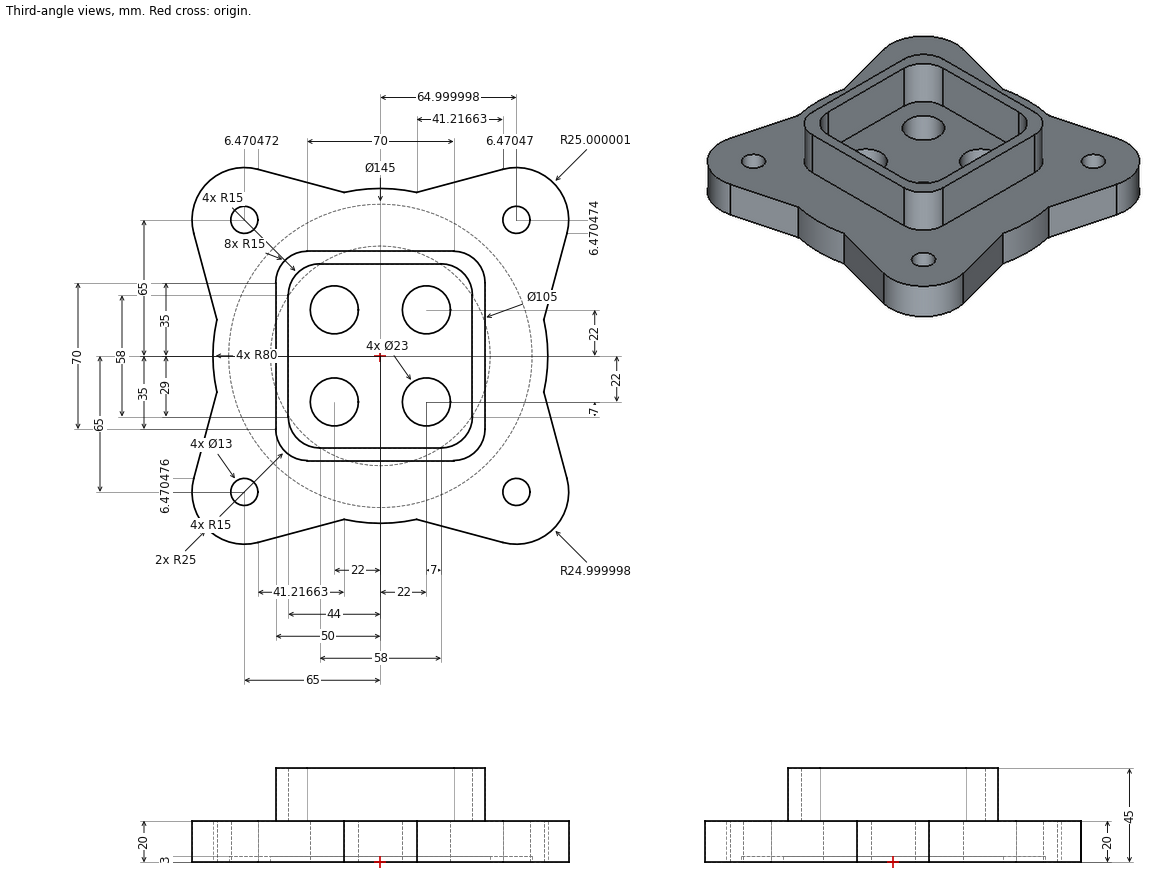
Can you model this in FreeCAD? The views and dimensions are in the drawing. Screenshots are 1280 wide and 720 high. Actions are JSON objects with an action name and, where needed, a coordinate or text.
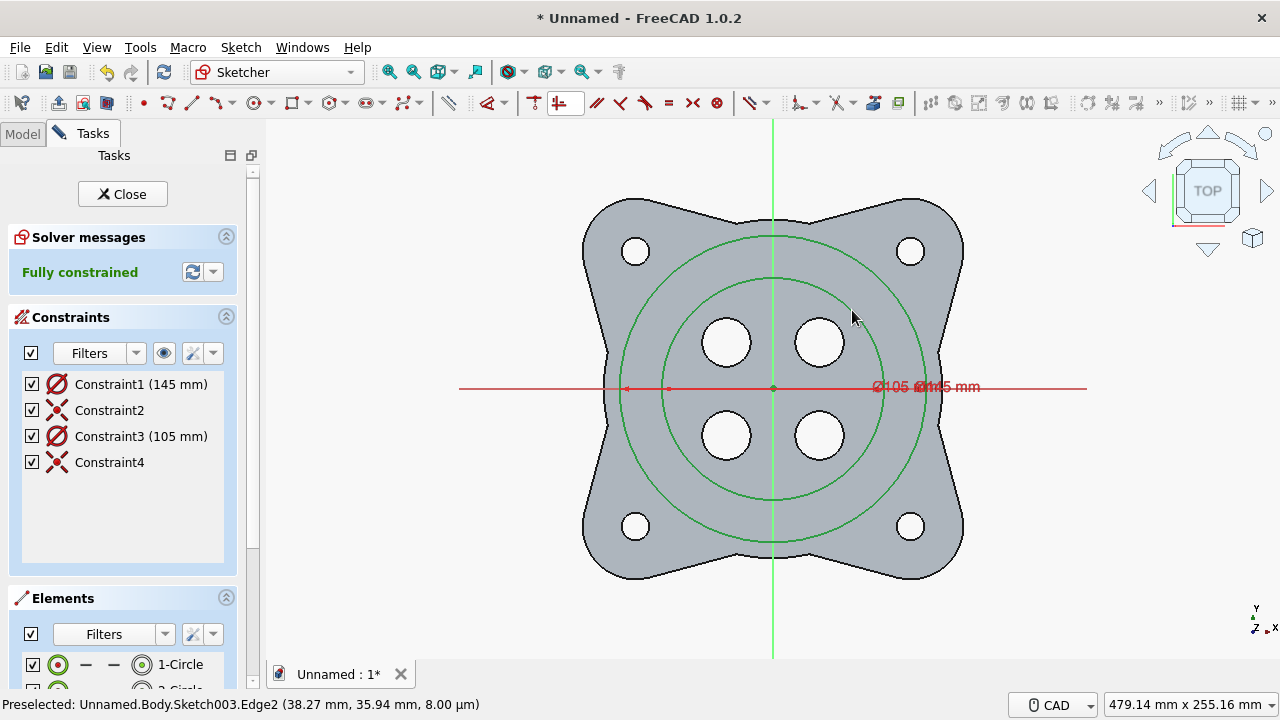
{"action": "left_click", "coordinate": [123, 194]}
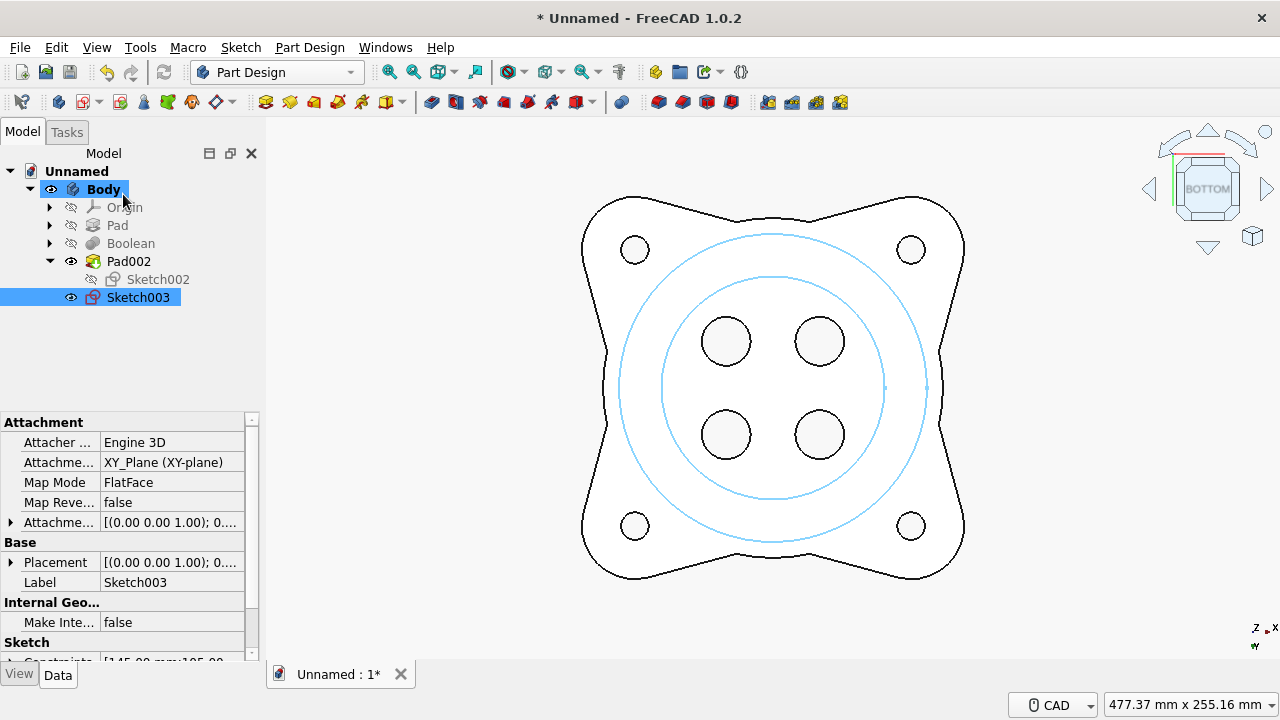
{"action": "left_click", "coordinate": [432, 102]}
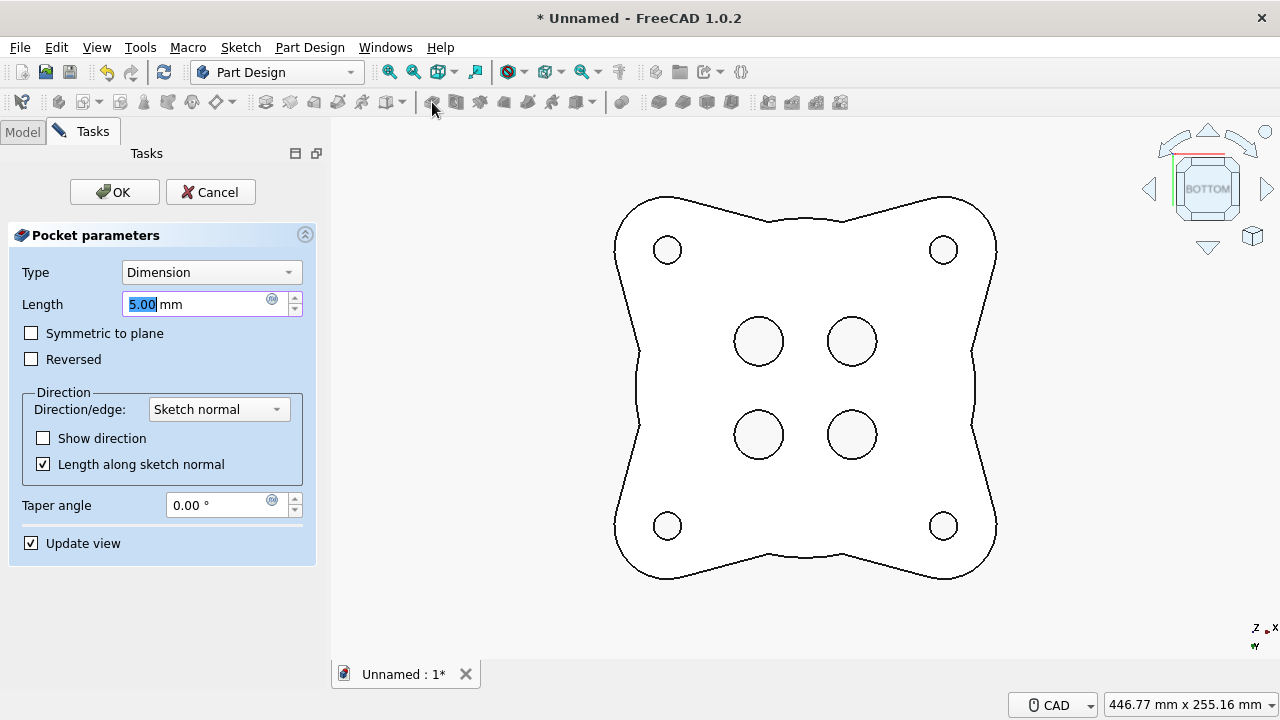
{"action": "type", "text": "3"}
{"action": "key", "text": "Tab"}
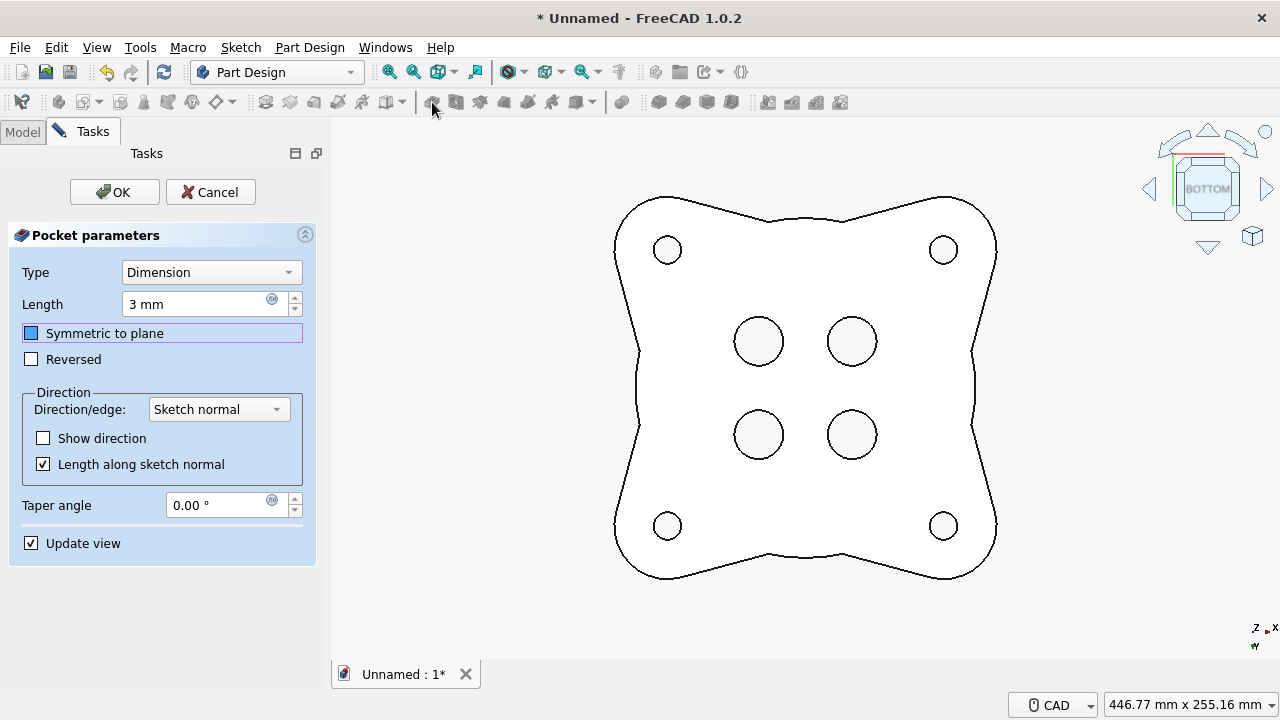
{"action": "left_click", "coordinate": [30, 359]}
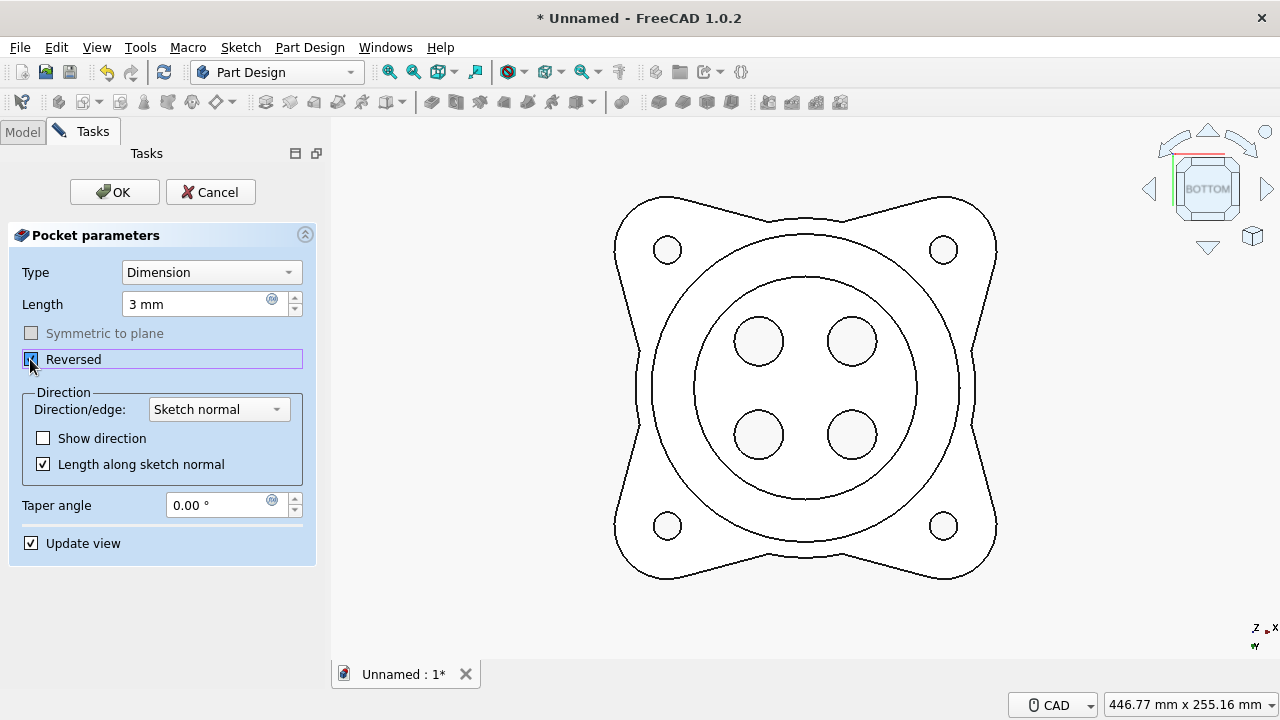
{"action": "left_click", "coordinate": [115, 192]}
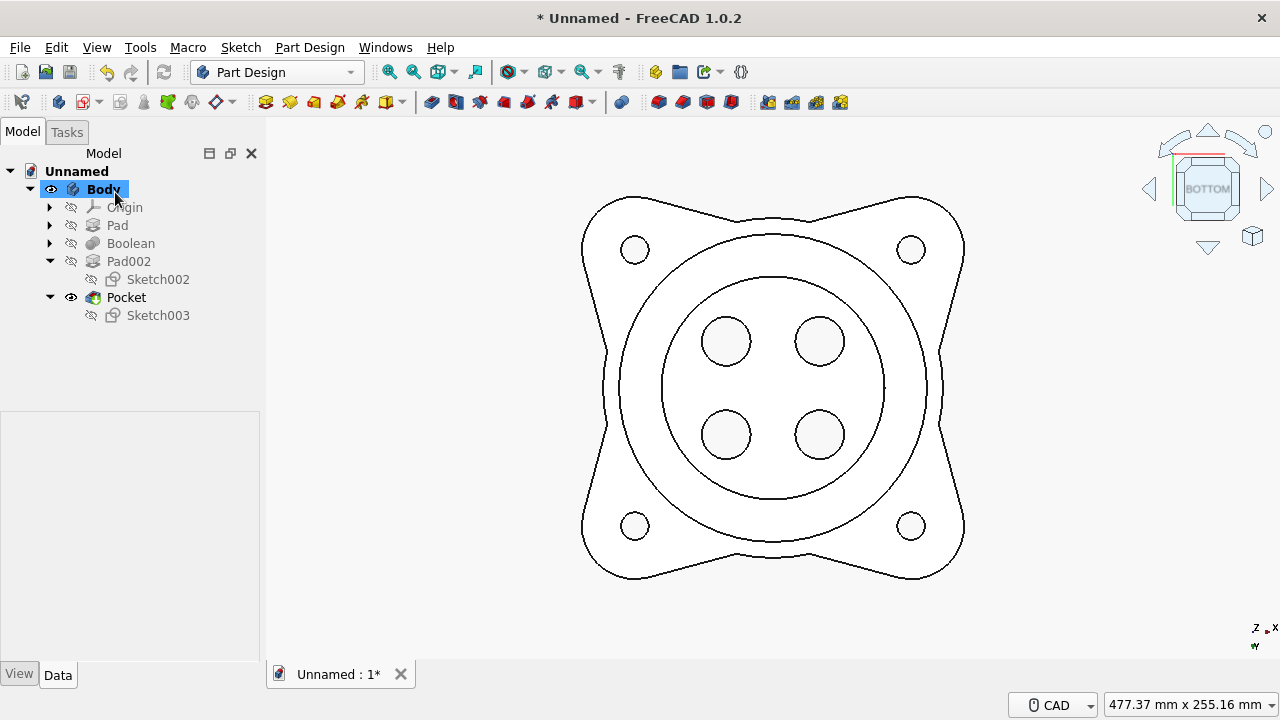
{"action": "key", "text": "0"}